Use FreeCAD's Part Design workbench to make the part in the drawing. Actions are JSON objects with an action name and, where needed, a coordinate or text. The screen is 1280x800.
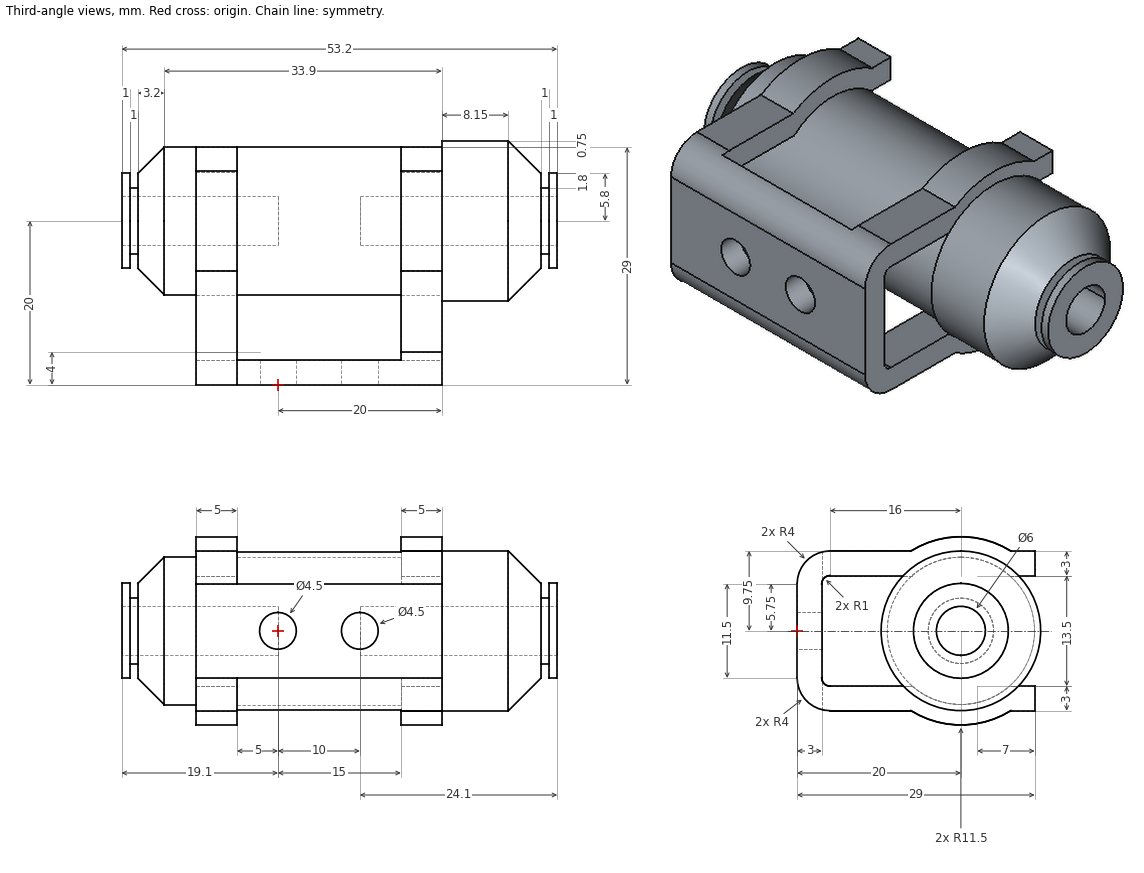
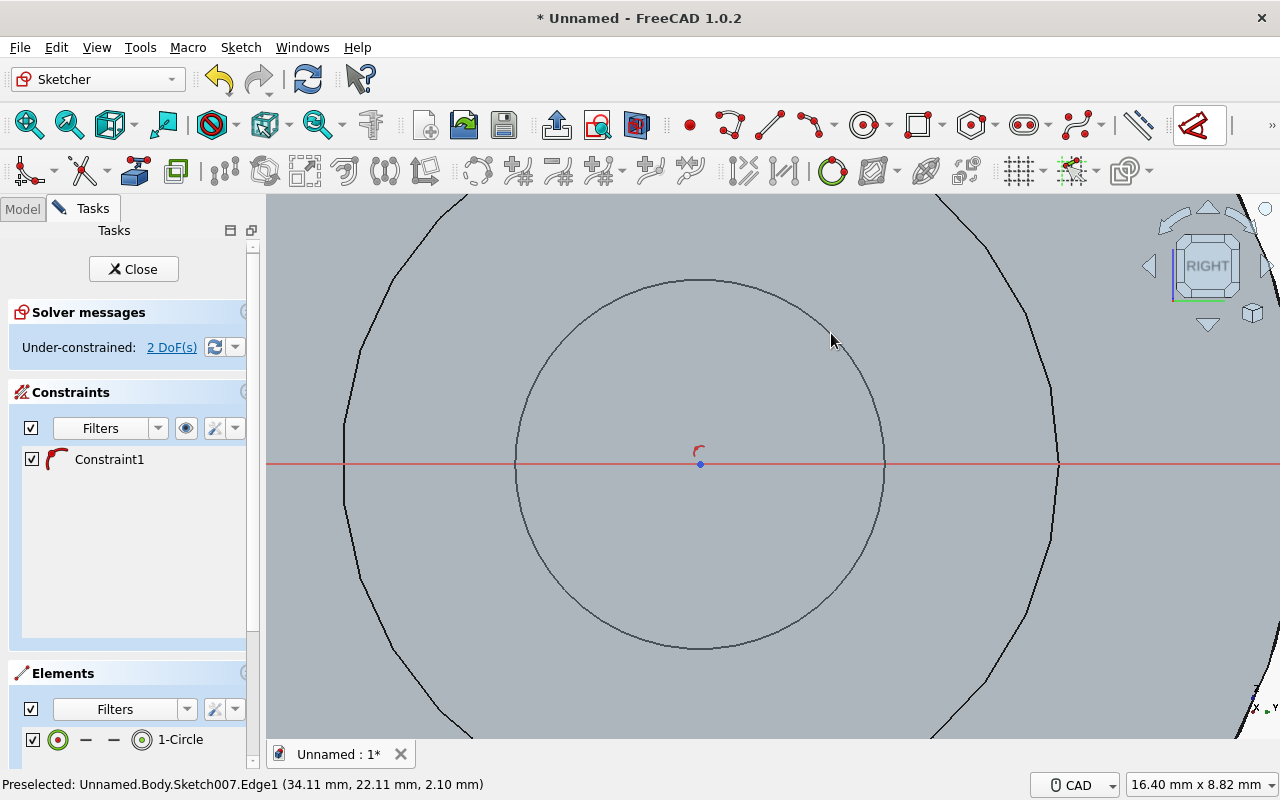
{"action": "left_click", "coordinate": [830, 333]}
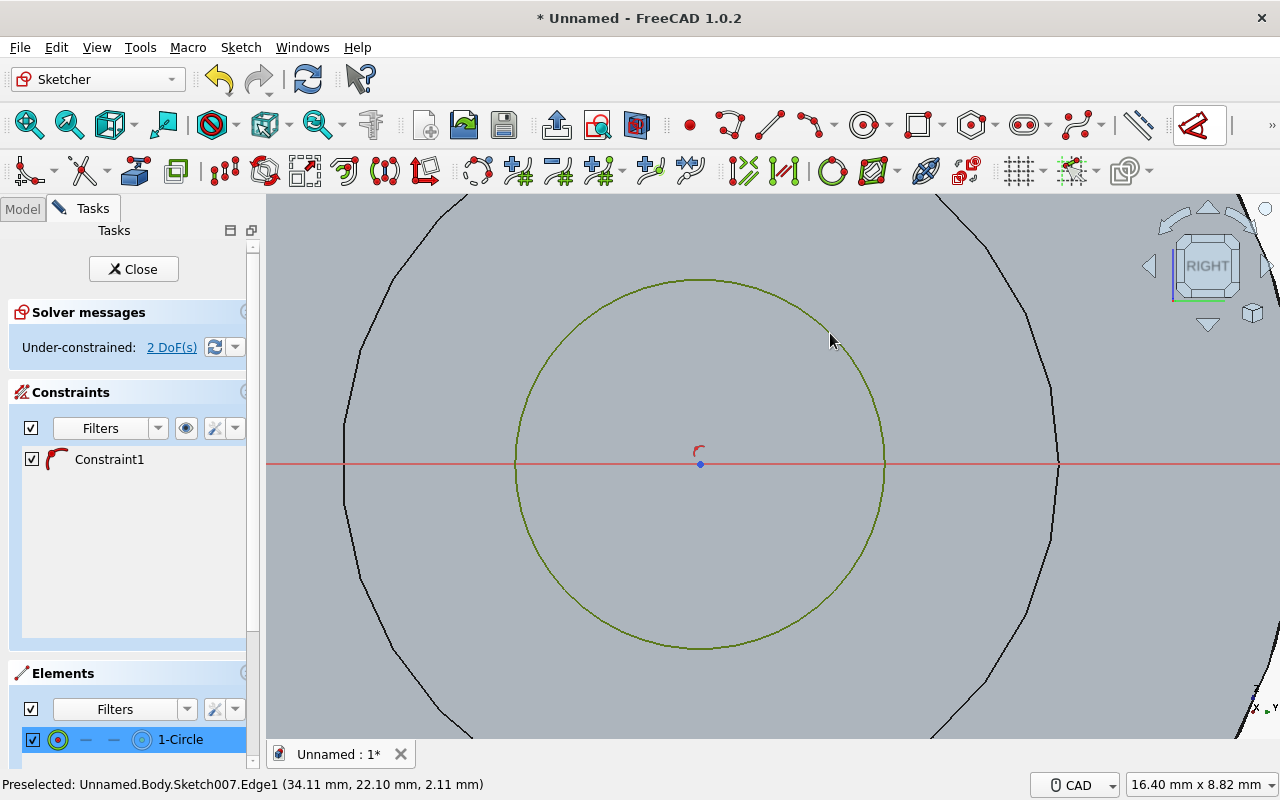
{"action": "left_click", "coordinate": [1220, 126]}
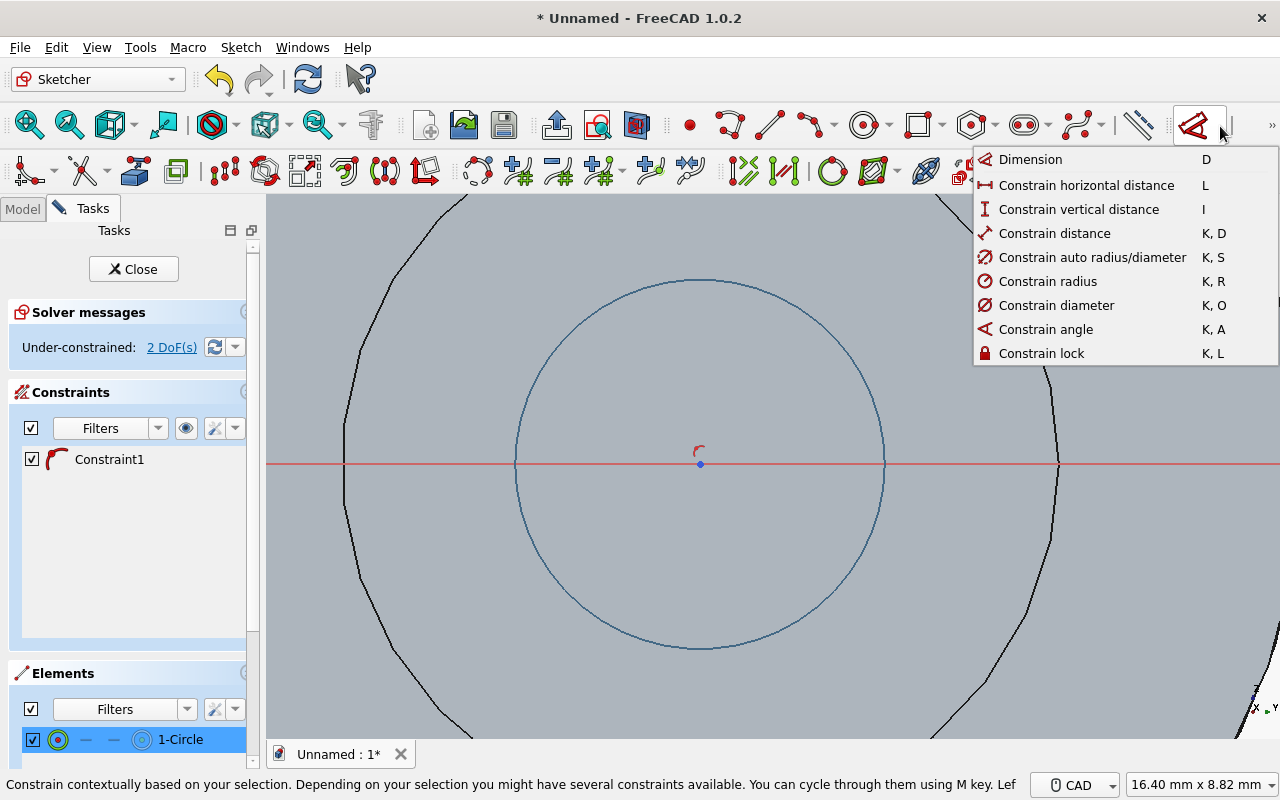
{"action": "left_click", "coordinate": [1126, 305]}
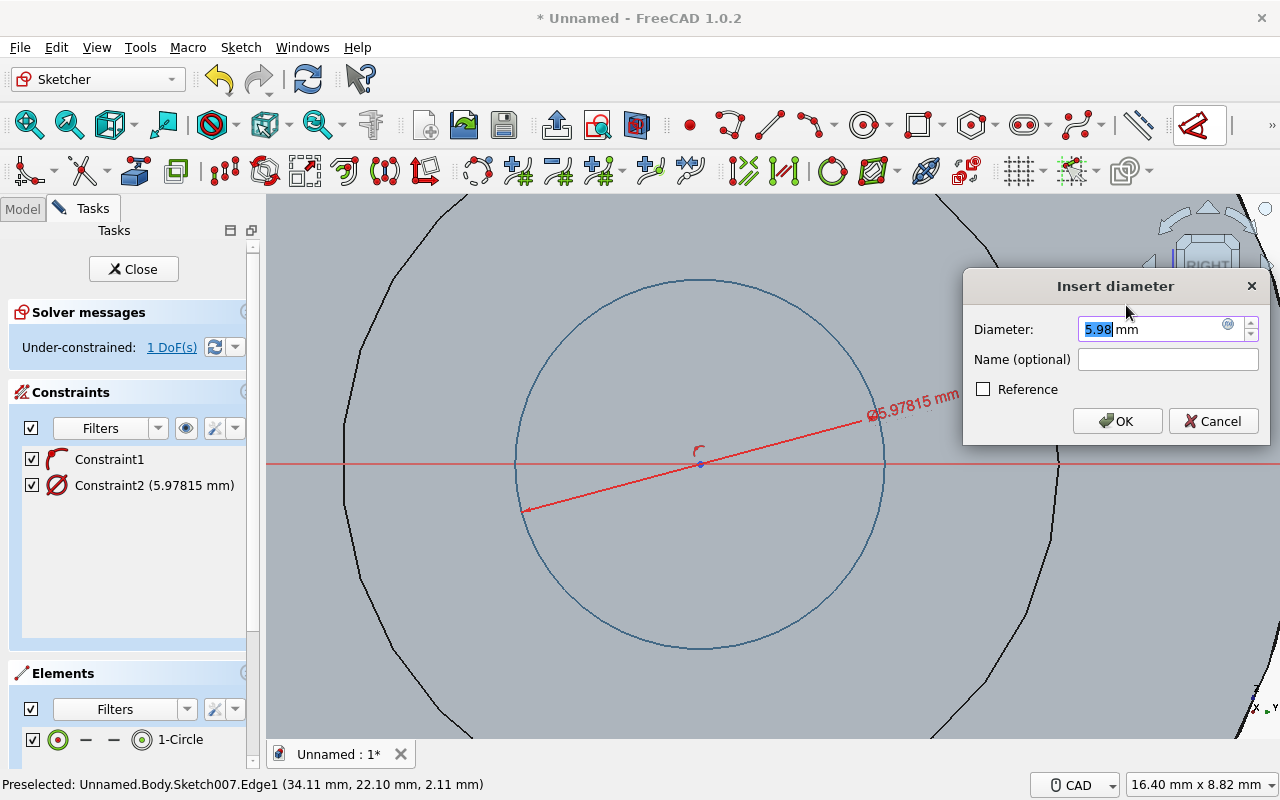
{"action": "type", "text": "6"}
{"action": "key", "text": "Return"}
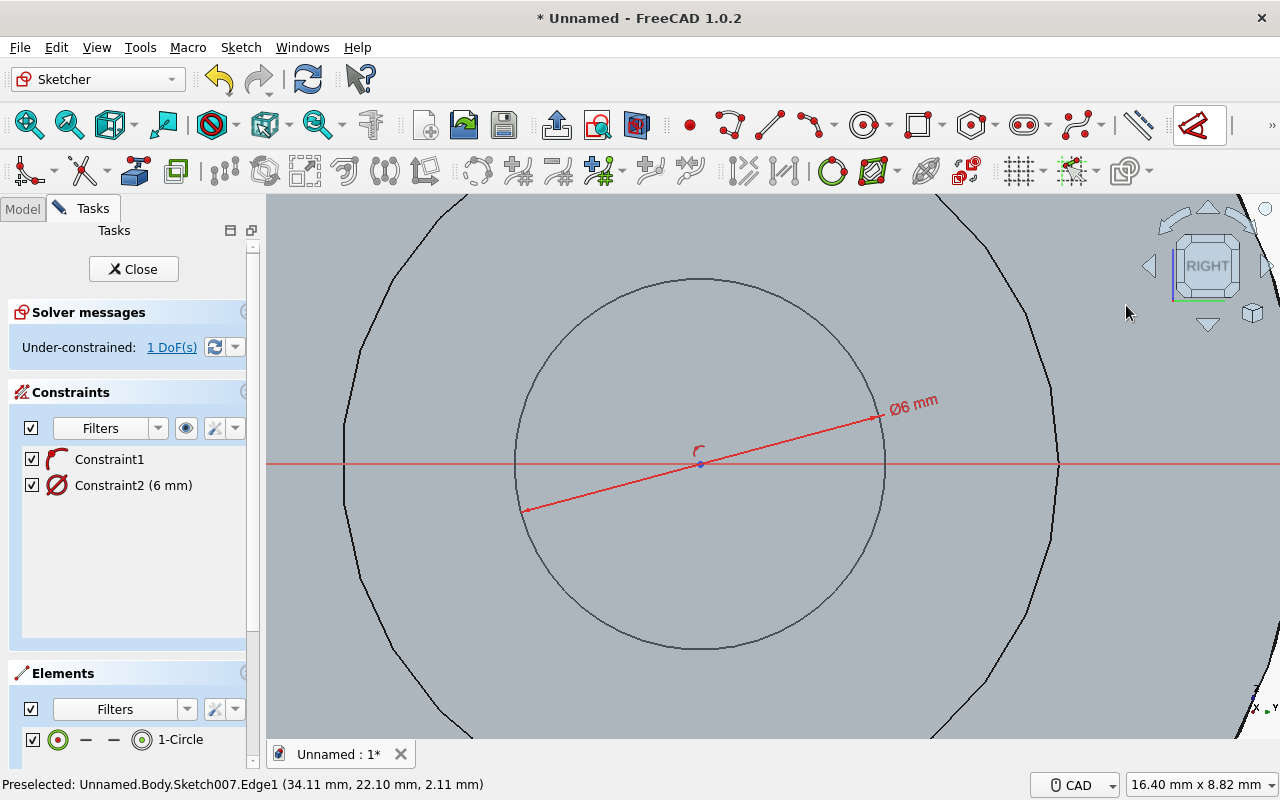
{"action": "left_click", "coordinate": [700, 464]}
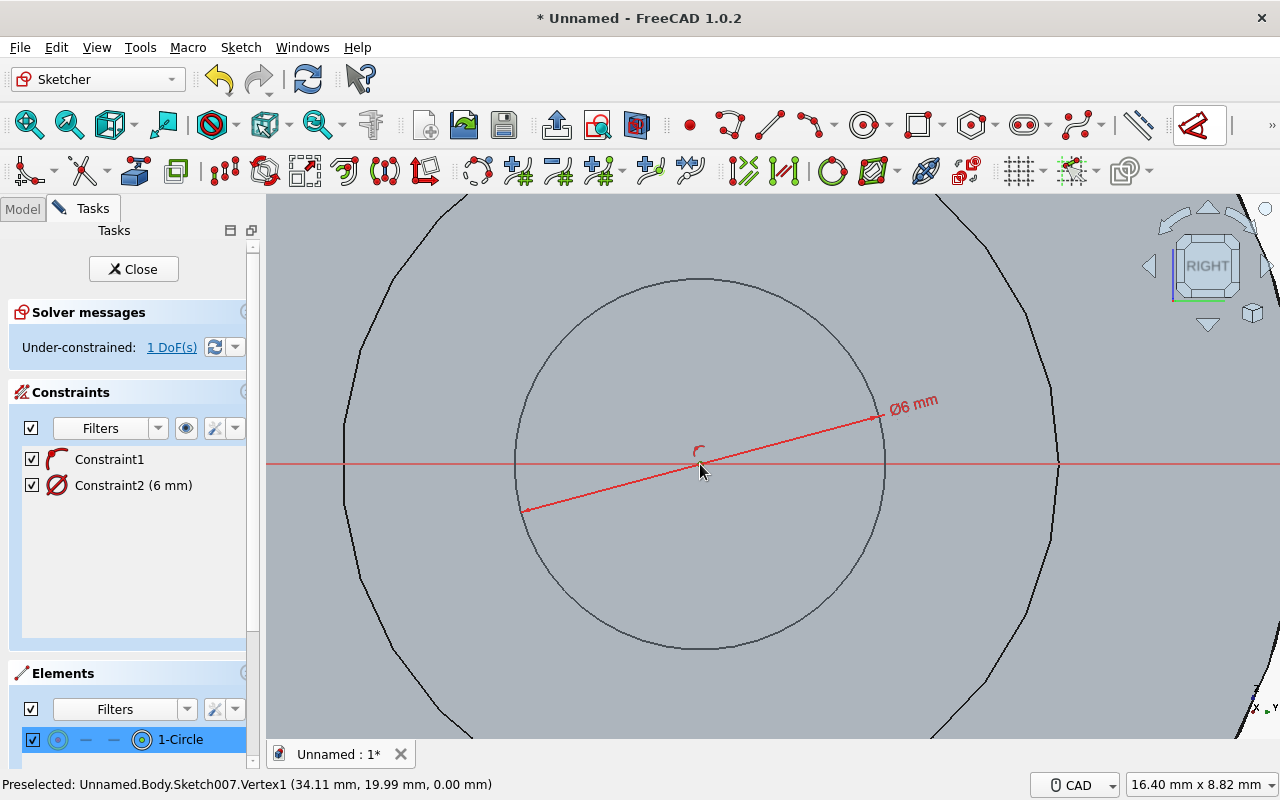
{"action": "key", "text": "l"}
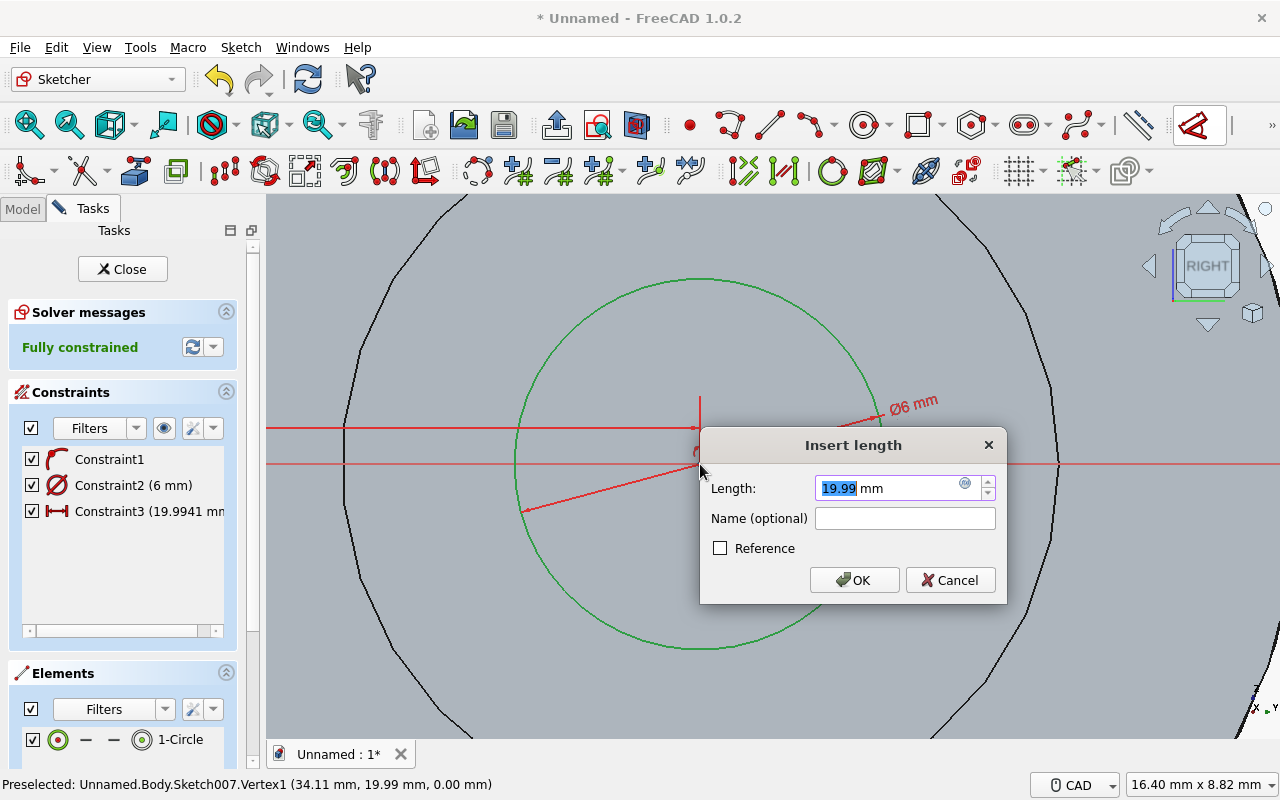
{"action": "type", "text": "20"}
{"action": "key", "text": "Return"}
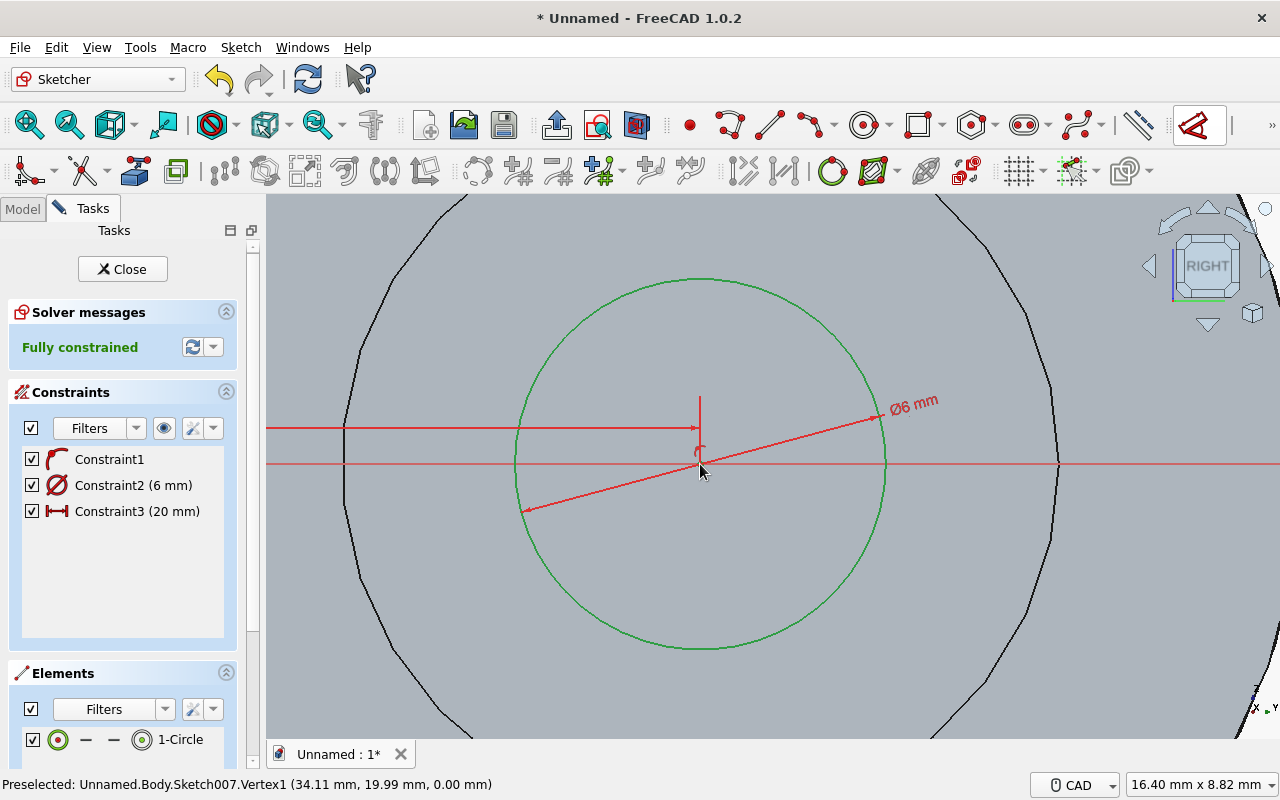
{"action": "left_click", "coordinate": [123, 269]}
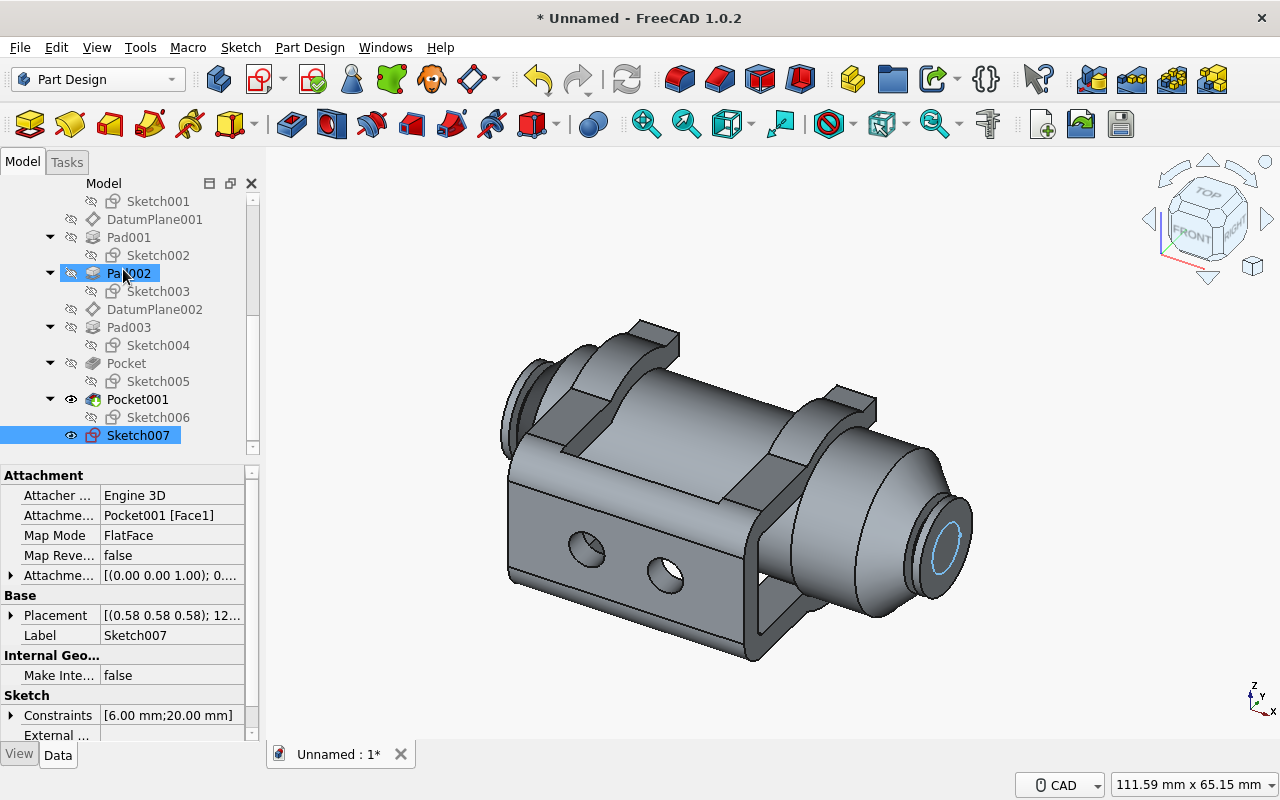
{"action": "left_click", "coordinate": [292, 124]}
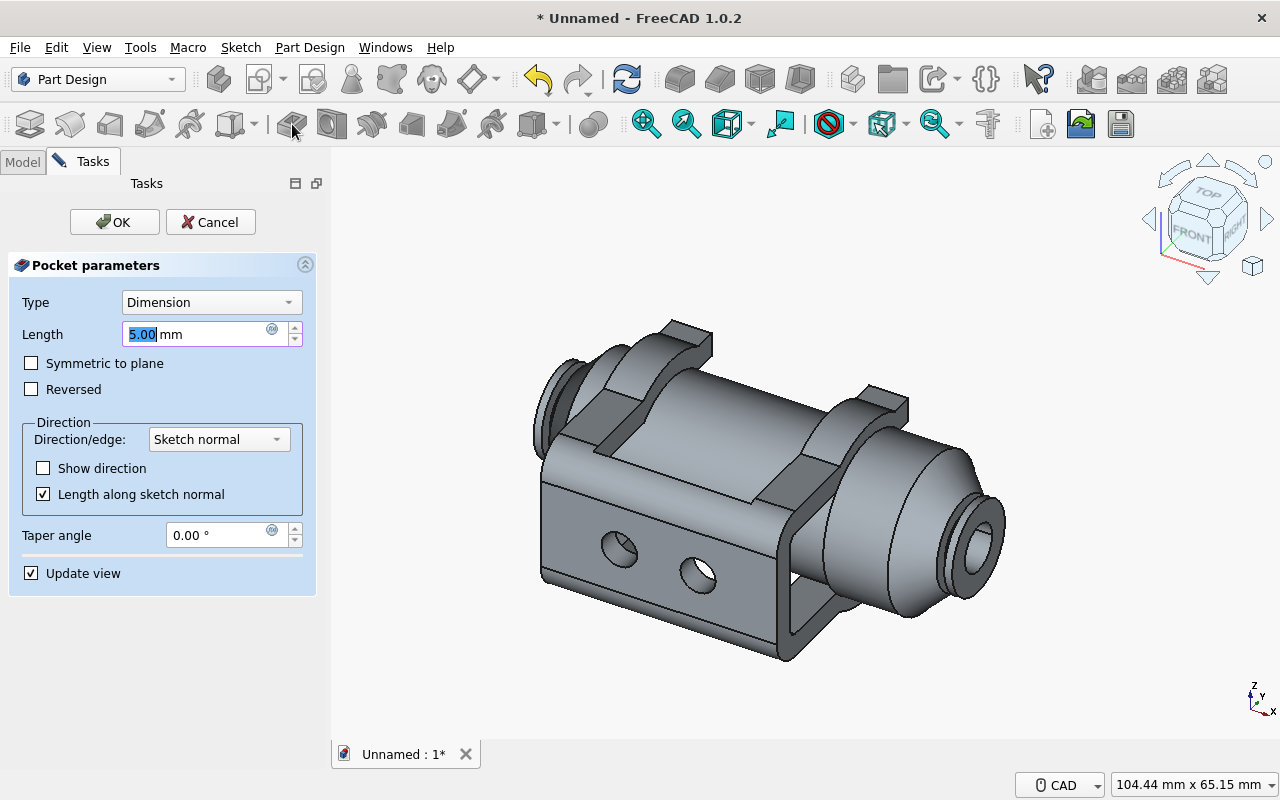
{"action": "type", "text": "24.1"}
{"action": "key", "text": "Tab"}